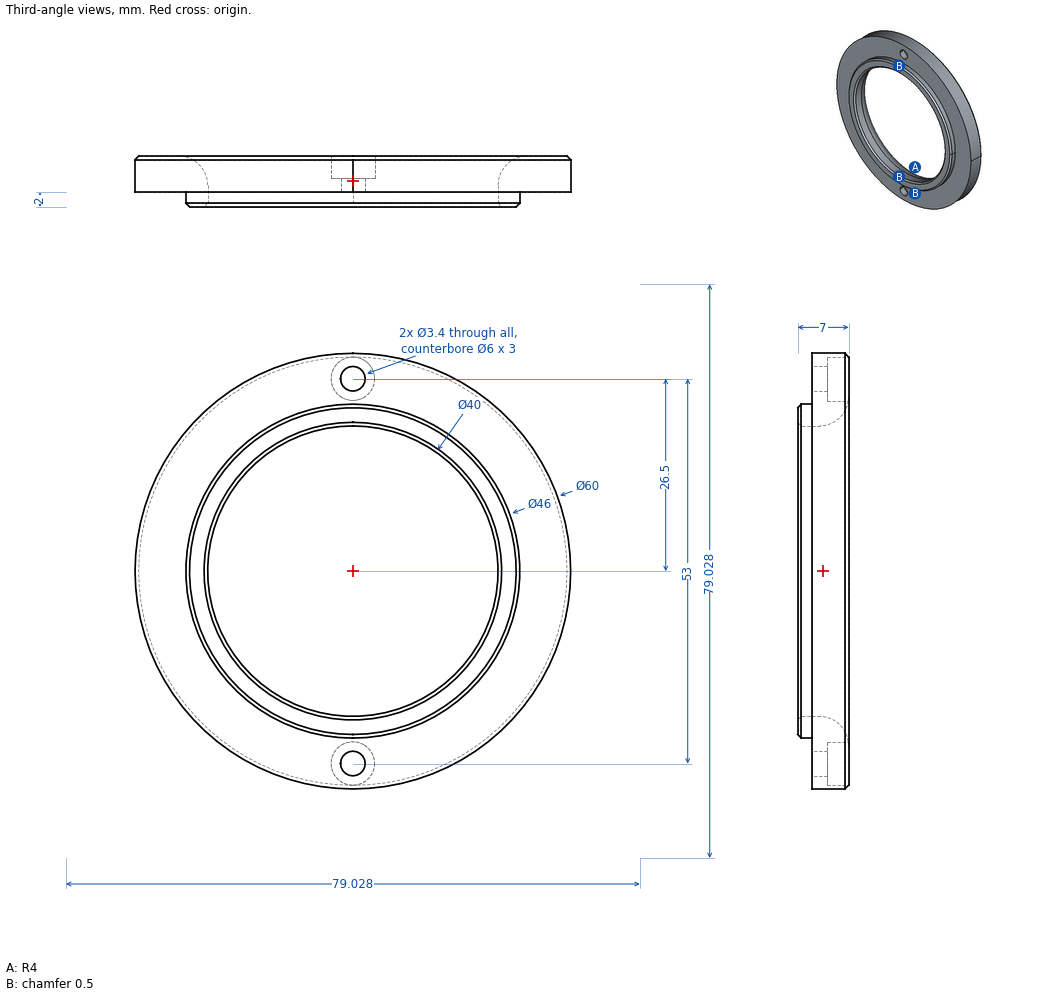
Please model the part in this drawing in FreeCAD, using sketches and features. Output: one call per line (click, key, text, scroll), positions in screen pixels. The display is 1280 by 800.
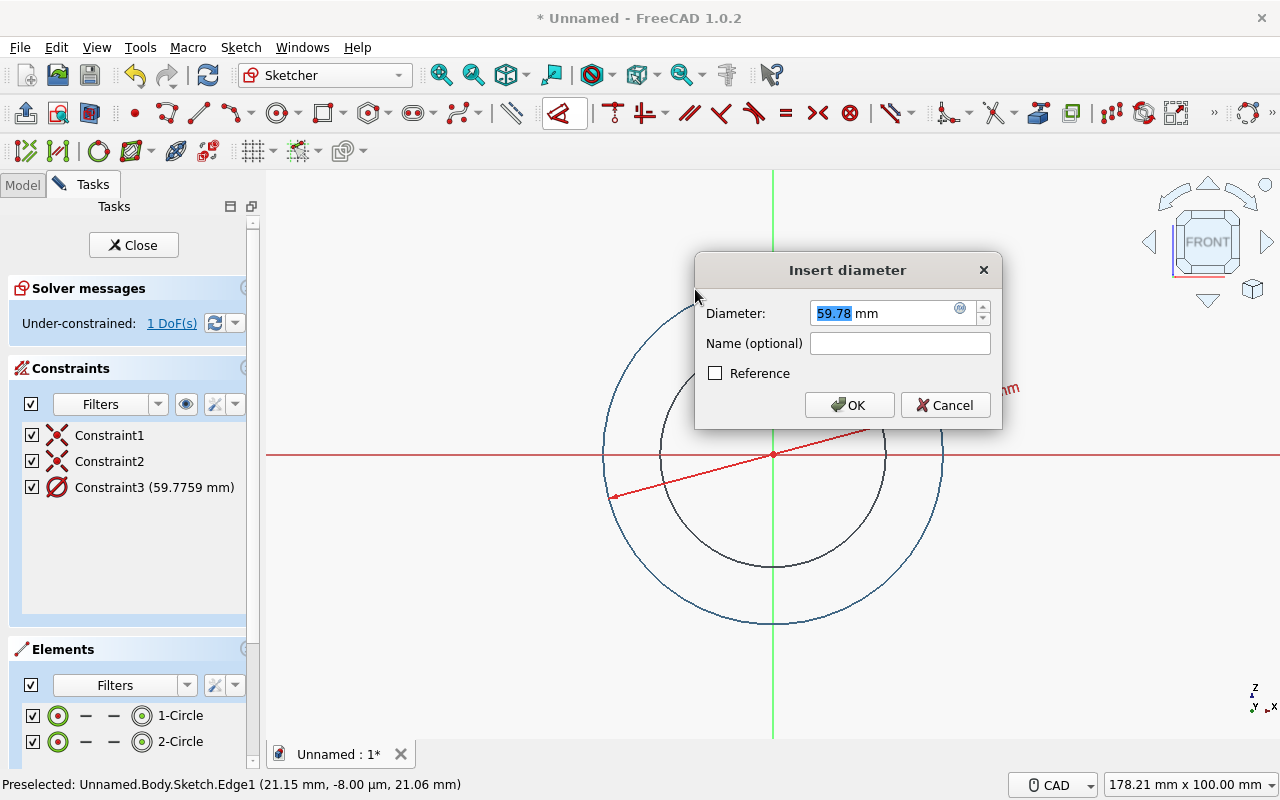
text(60)
key(Return)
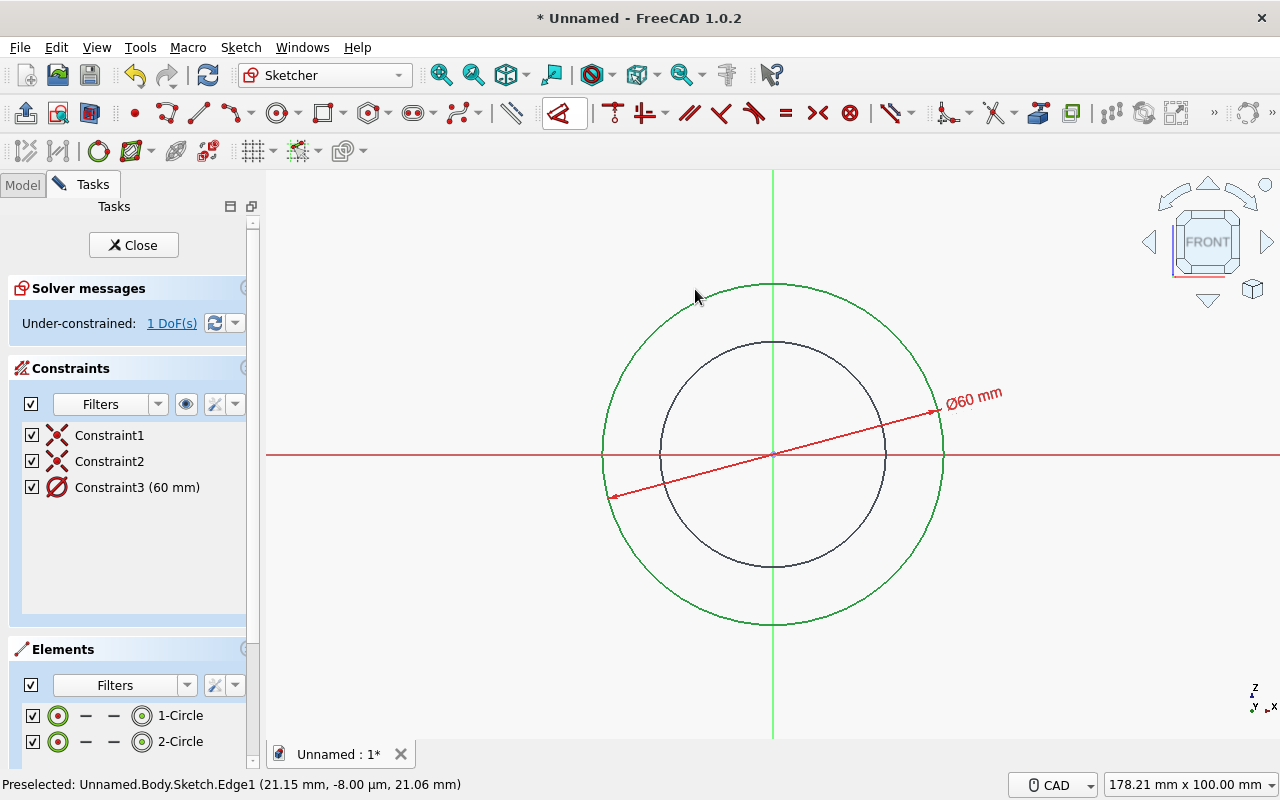
click(853, 375)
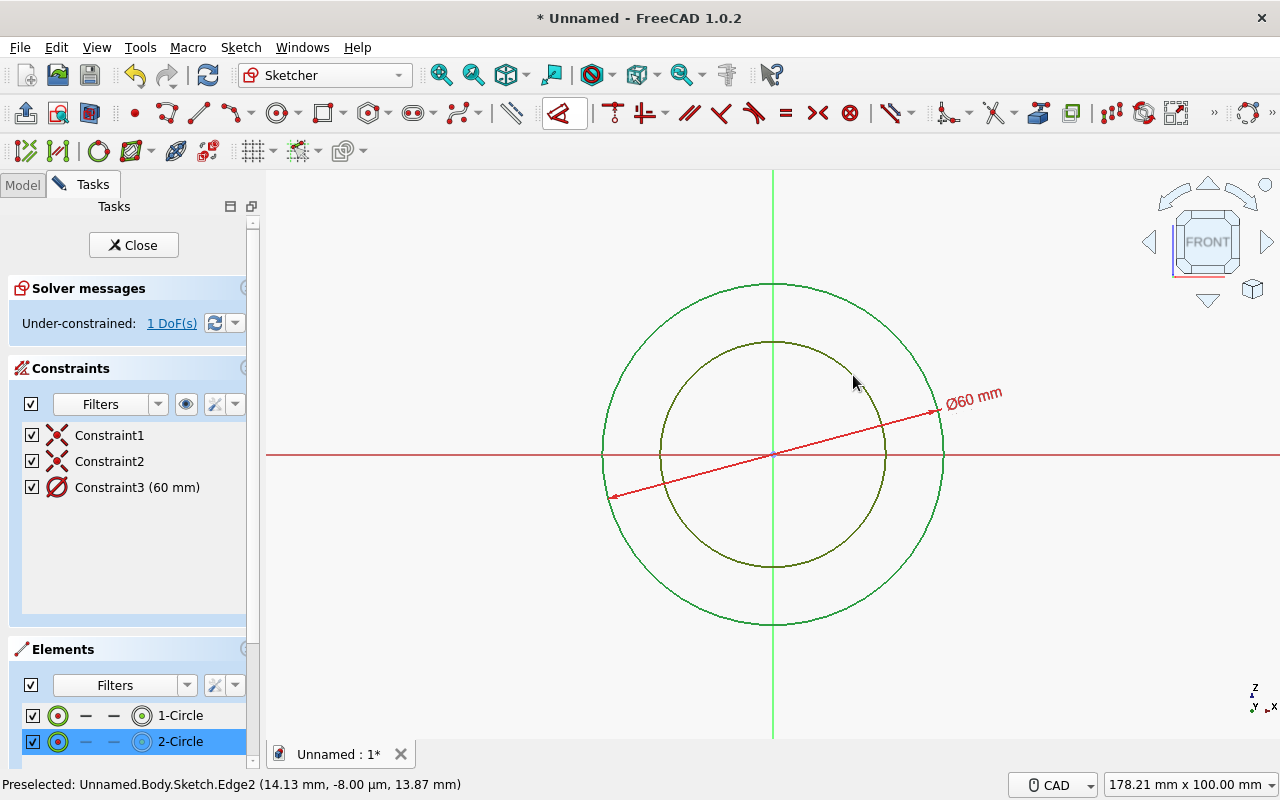
key(k)
key(o)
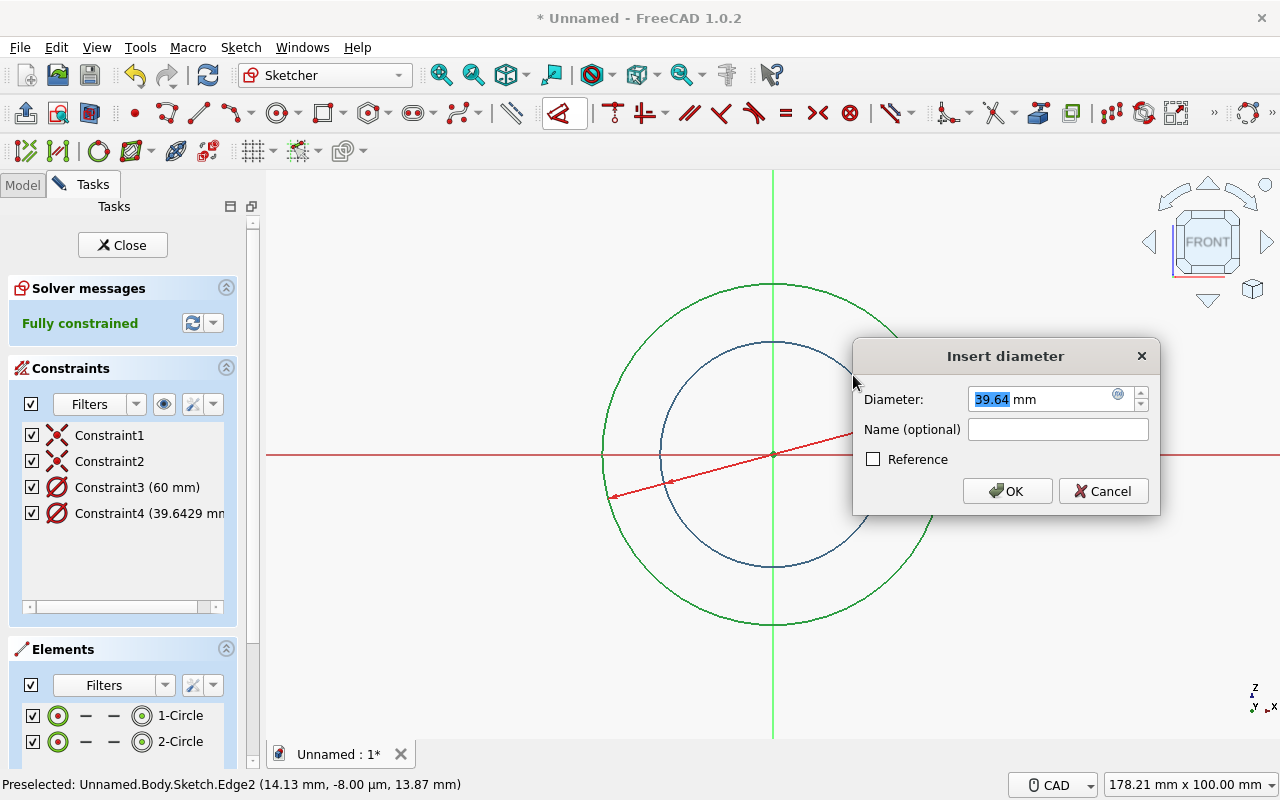
text(40)
key(Return)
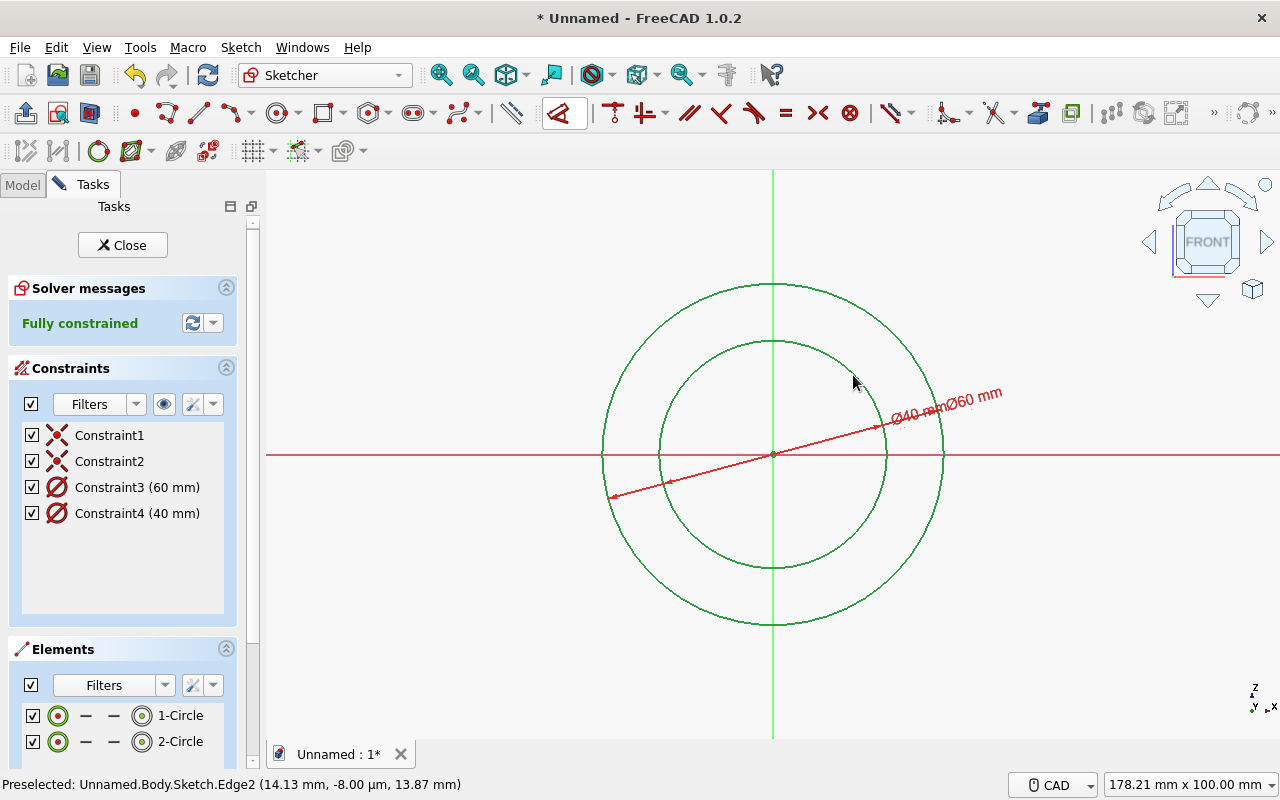
click(123, 245)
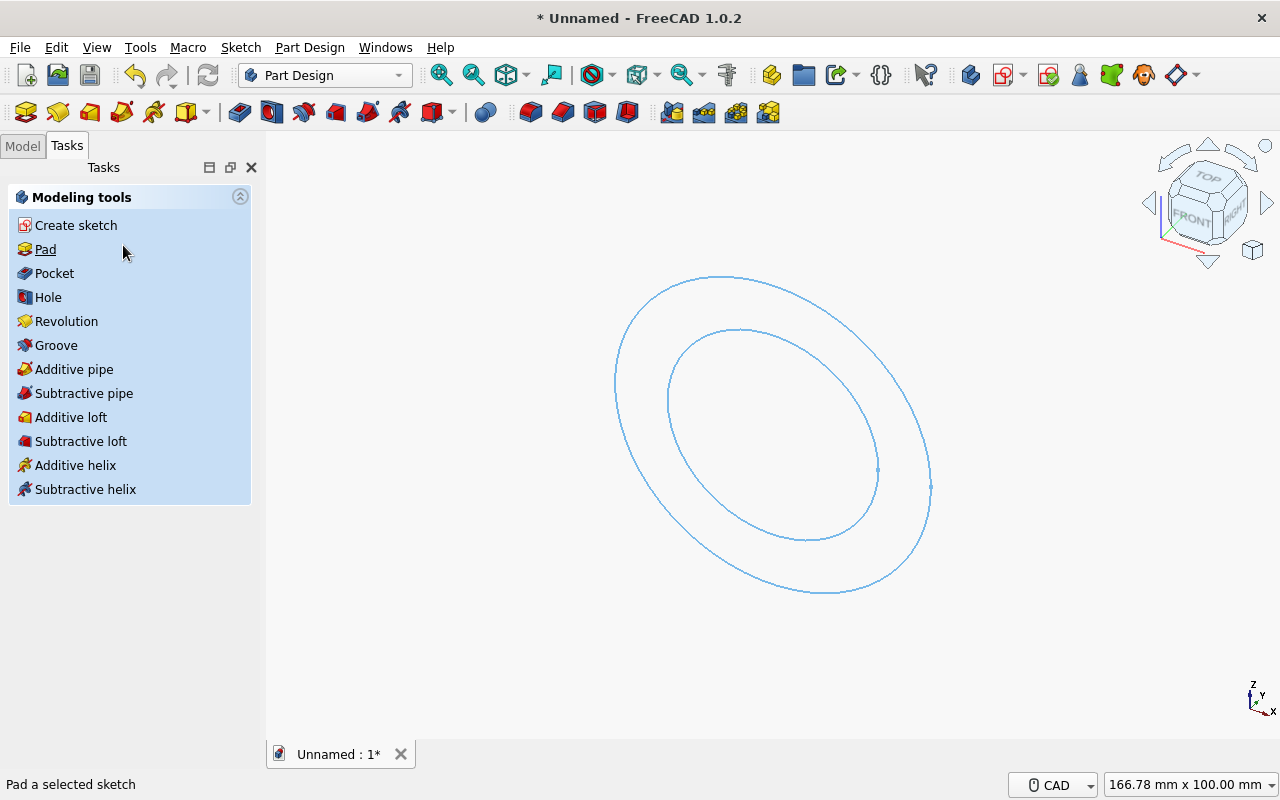
click(26, 112)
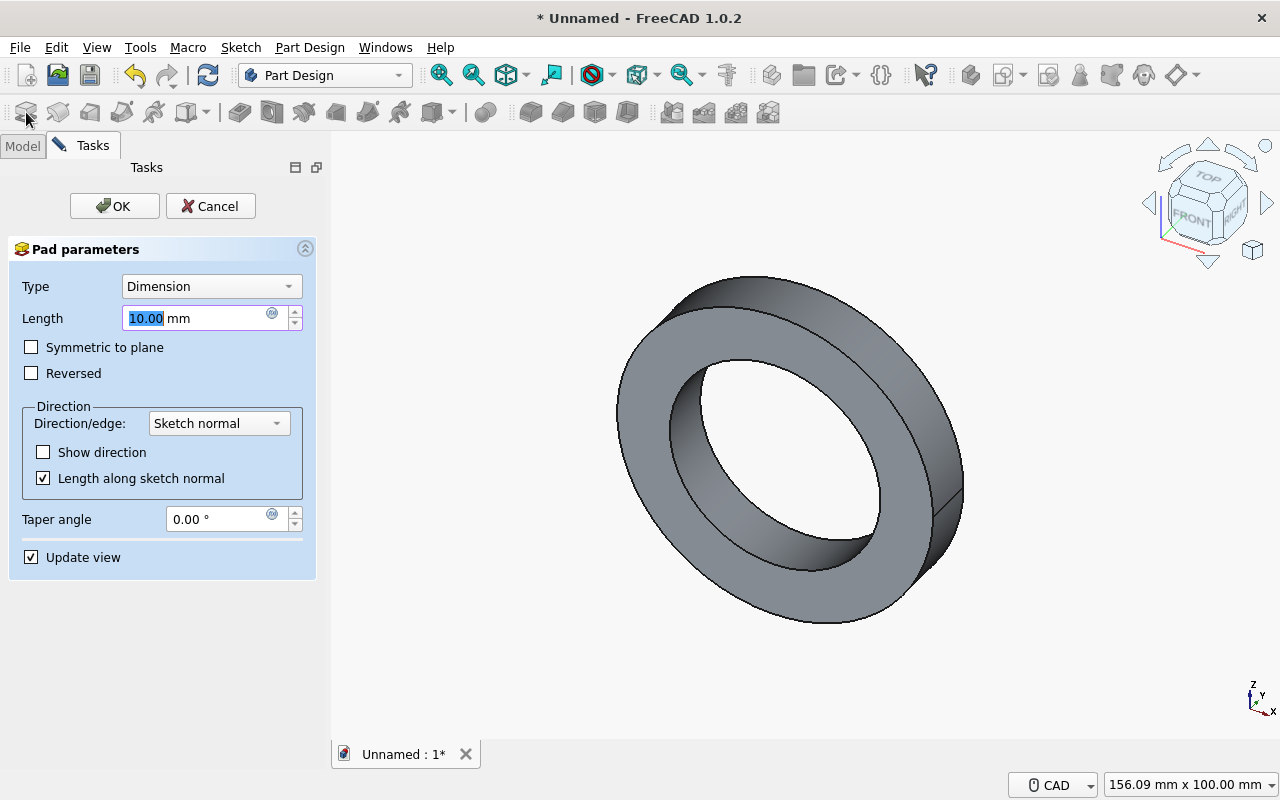
text(7)
key(Tab)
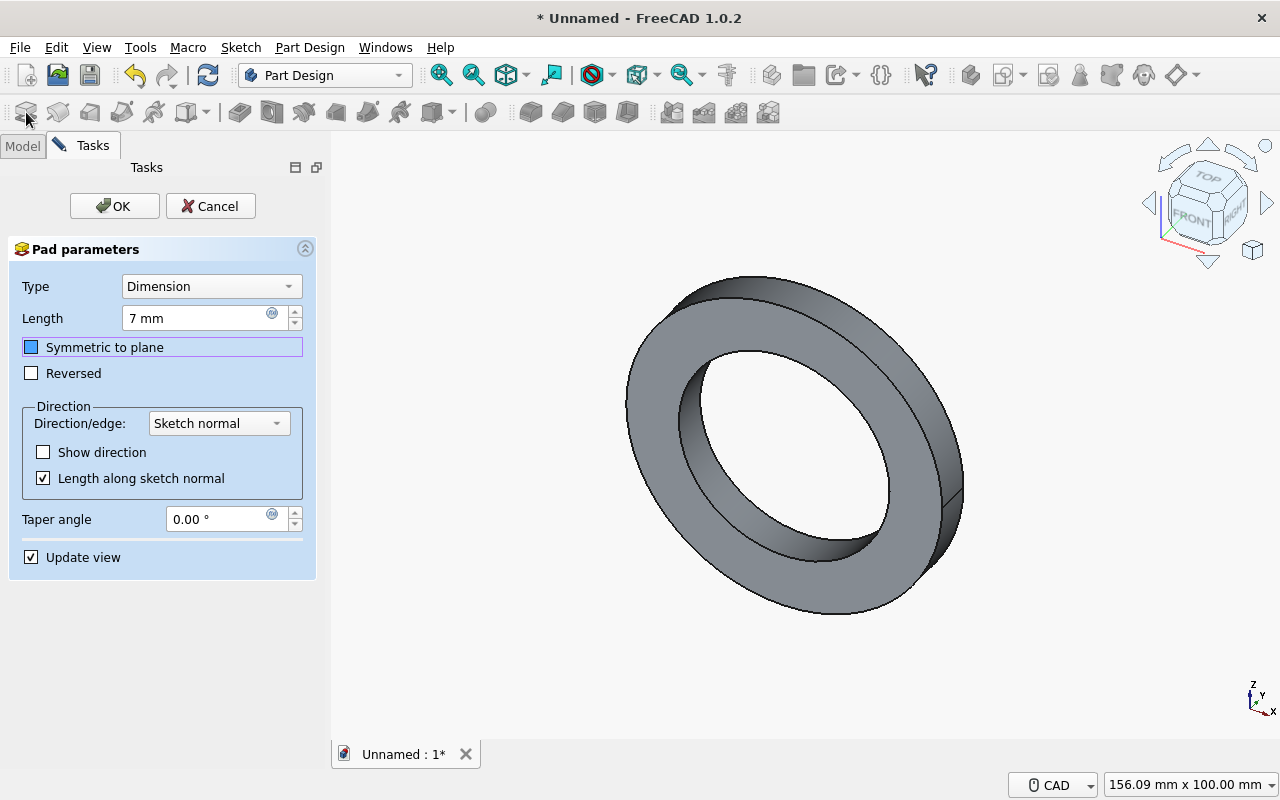
click(30, 347)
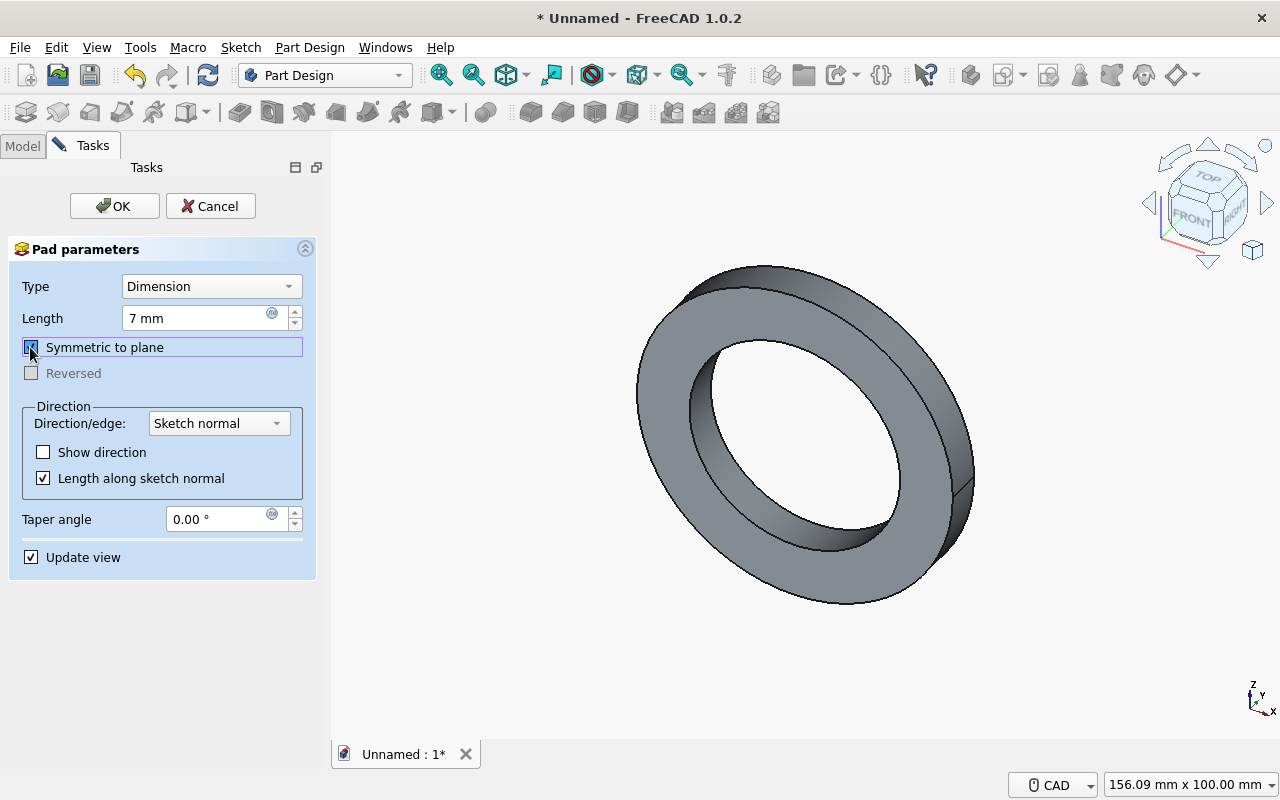
click(115, 206)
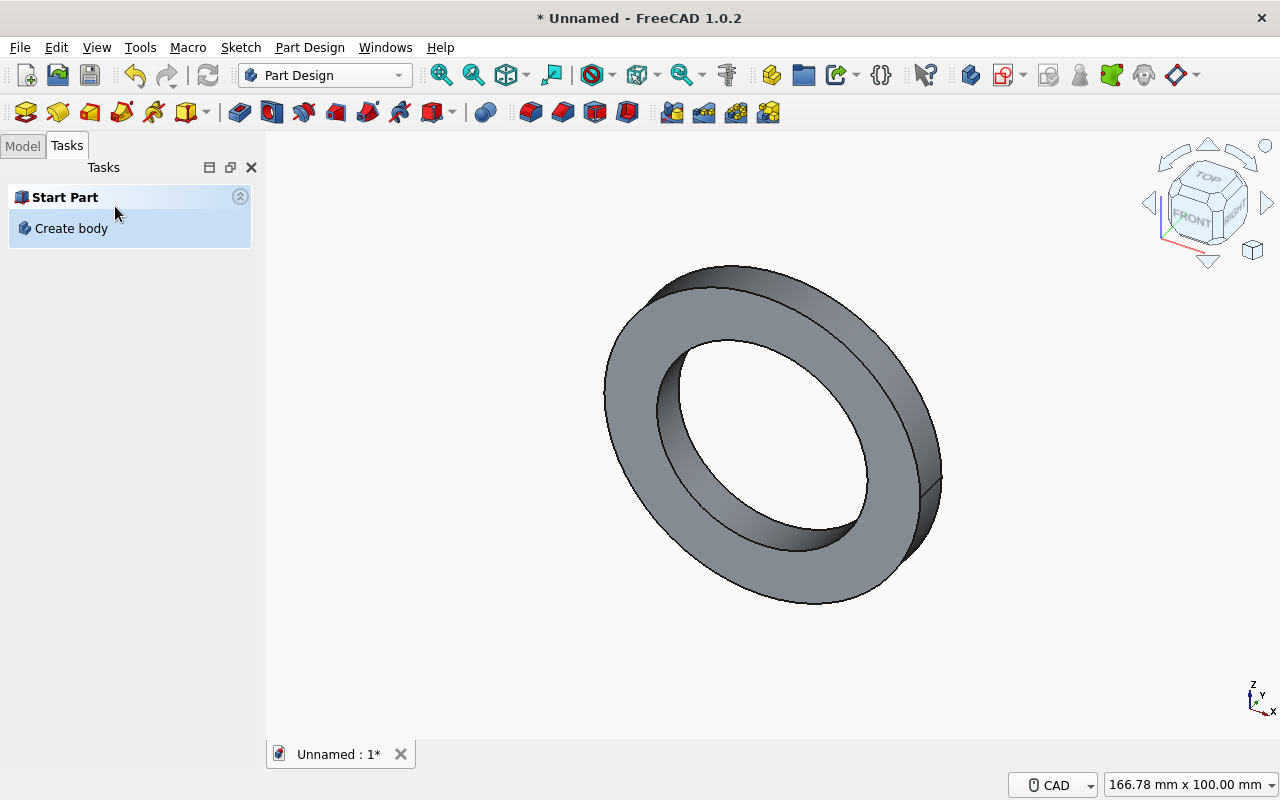
click(898, 489)